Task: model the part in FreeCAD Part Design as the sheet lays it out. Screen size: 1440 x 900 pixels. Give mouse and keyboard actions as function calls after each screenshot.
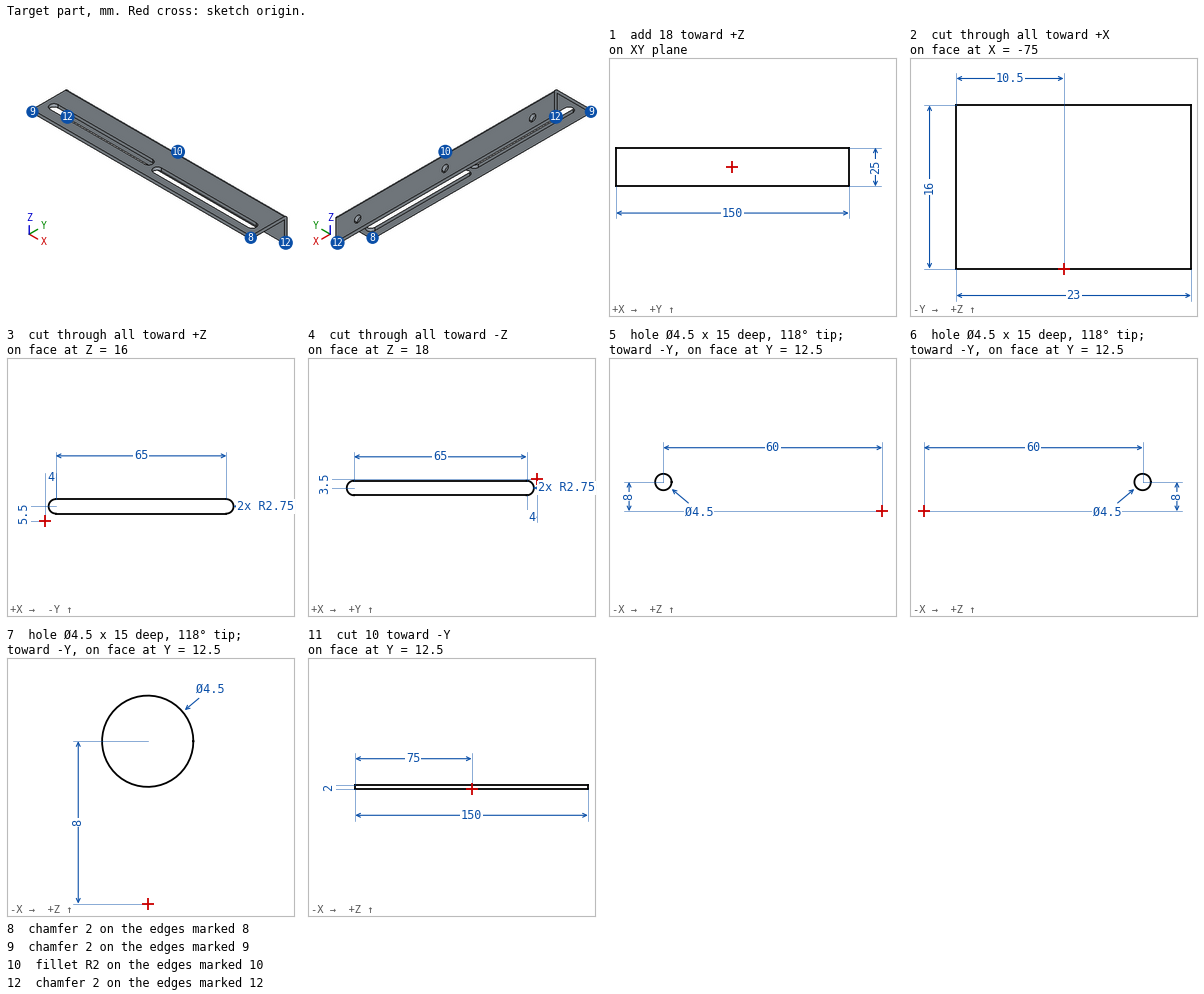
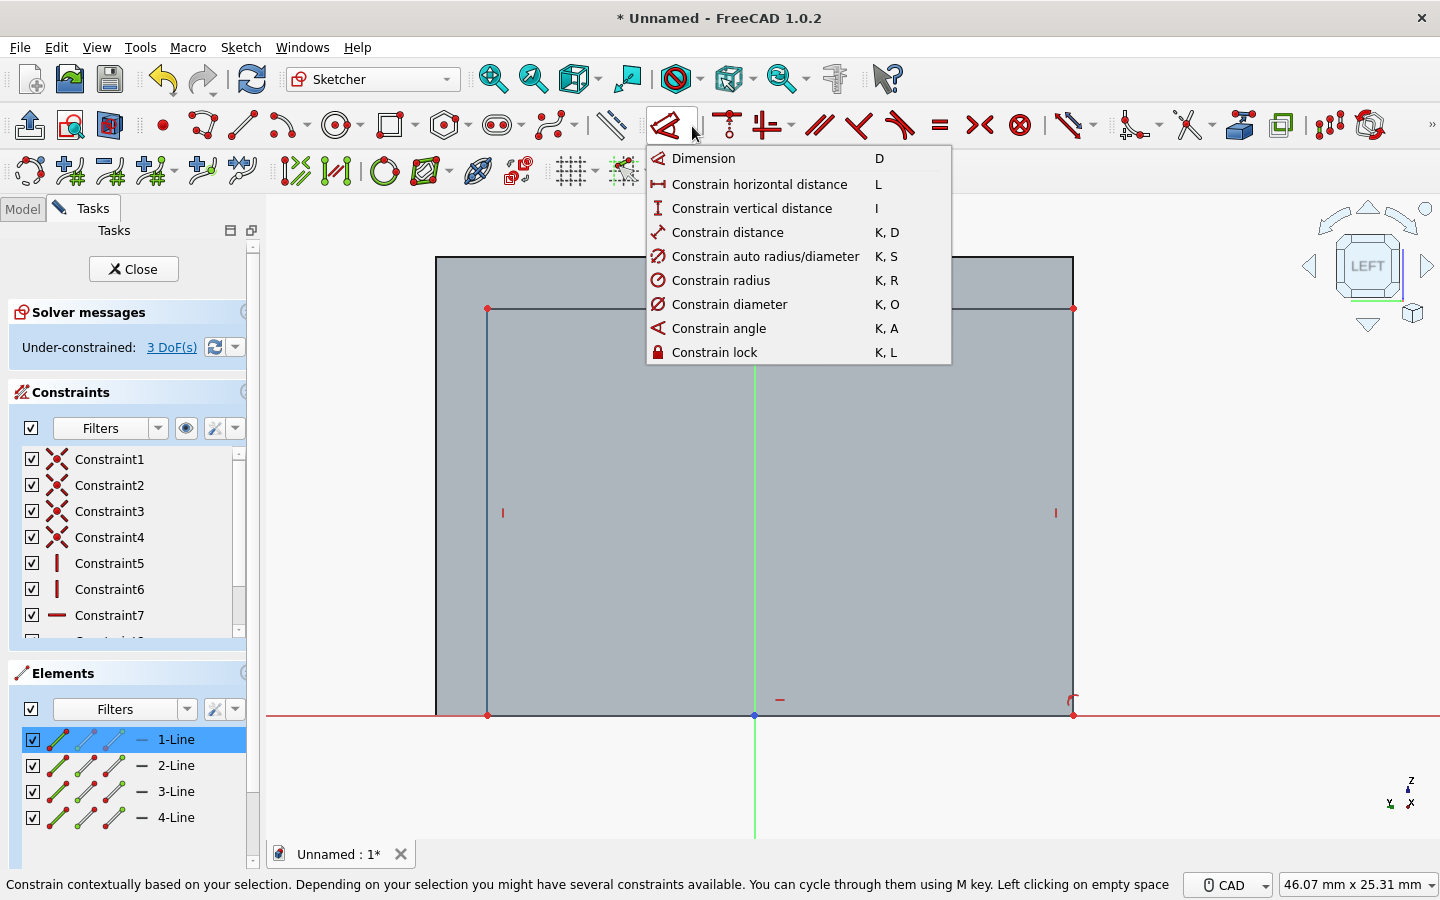
click(799, 208)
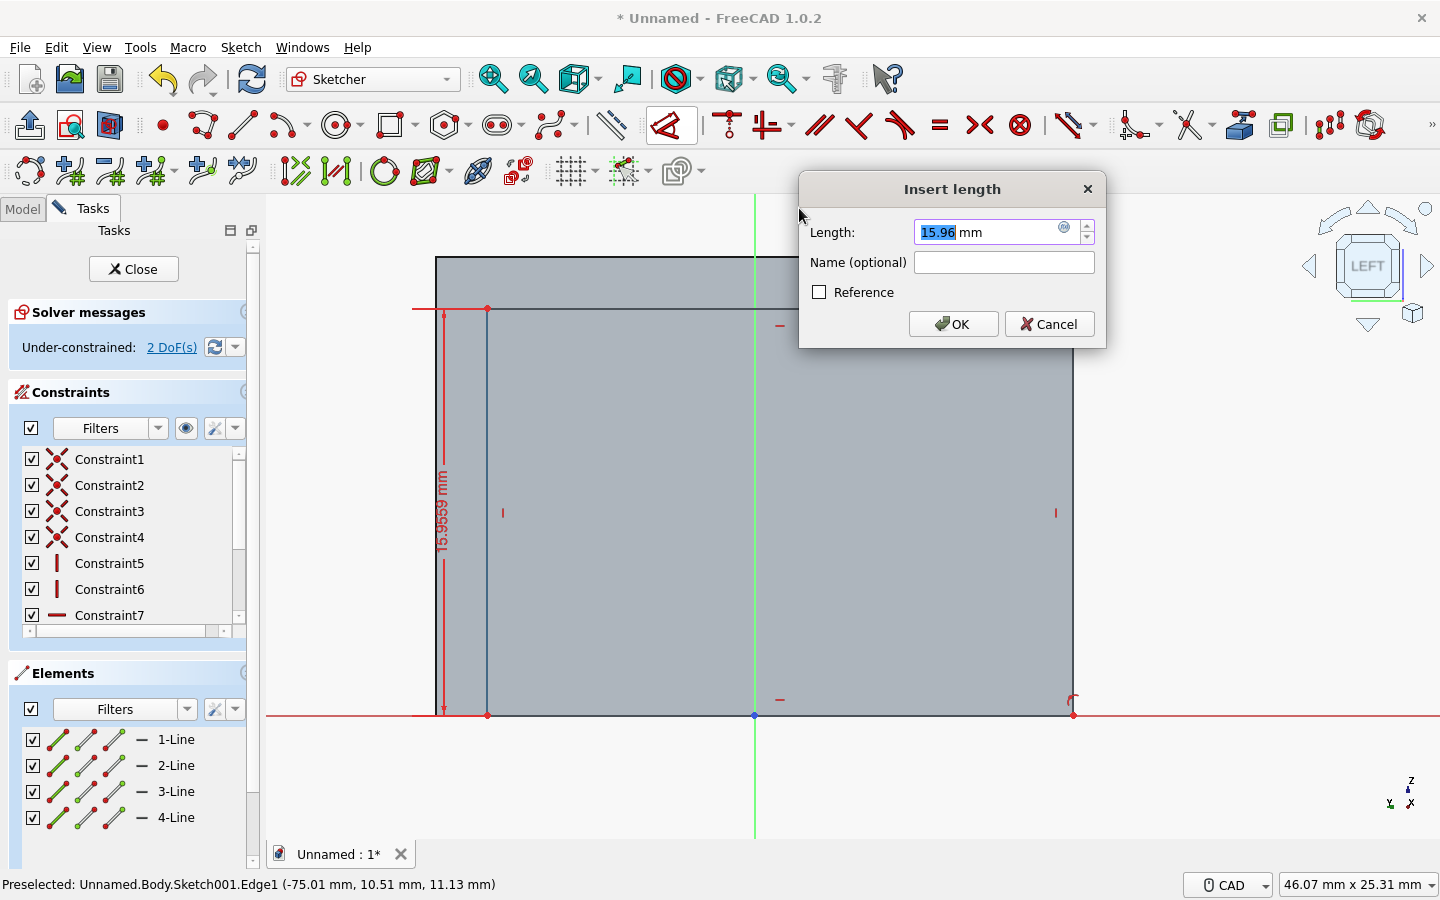
text(16)
key(Return)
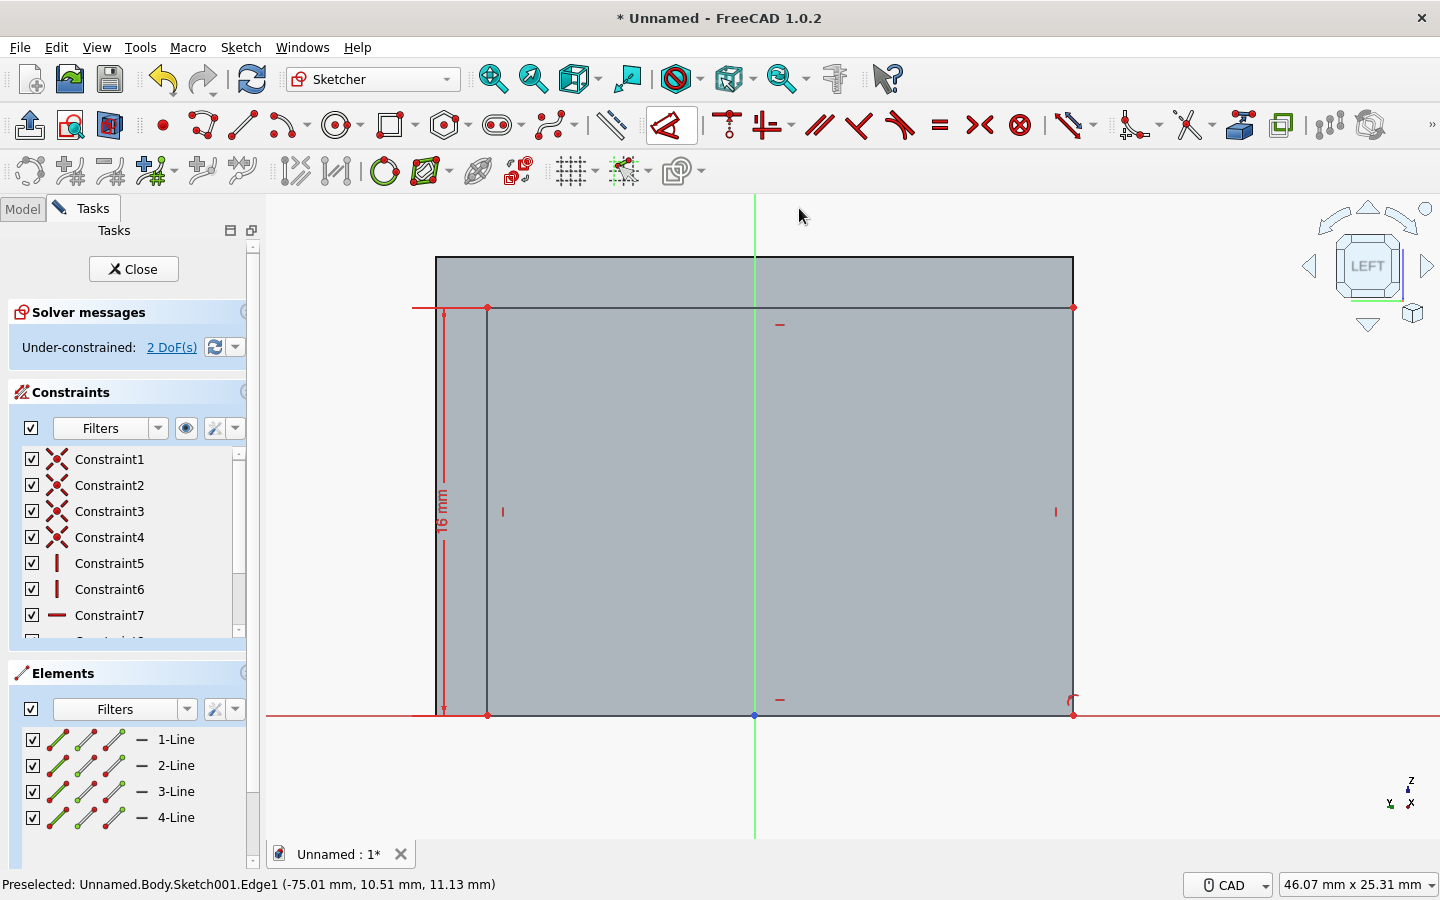
click(663, 716)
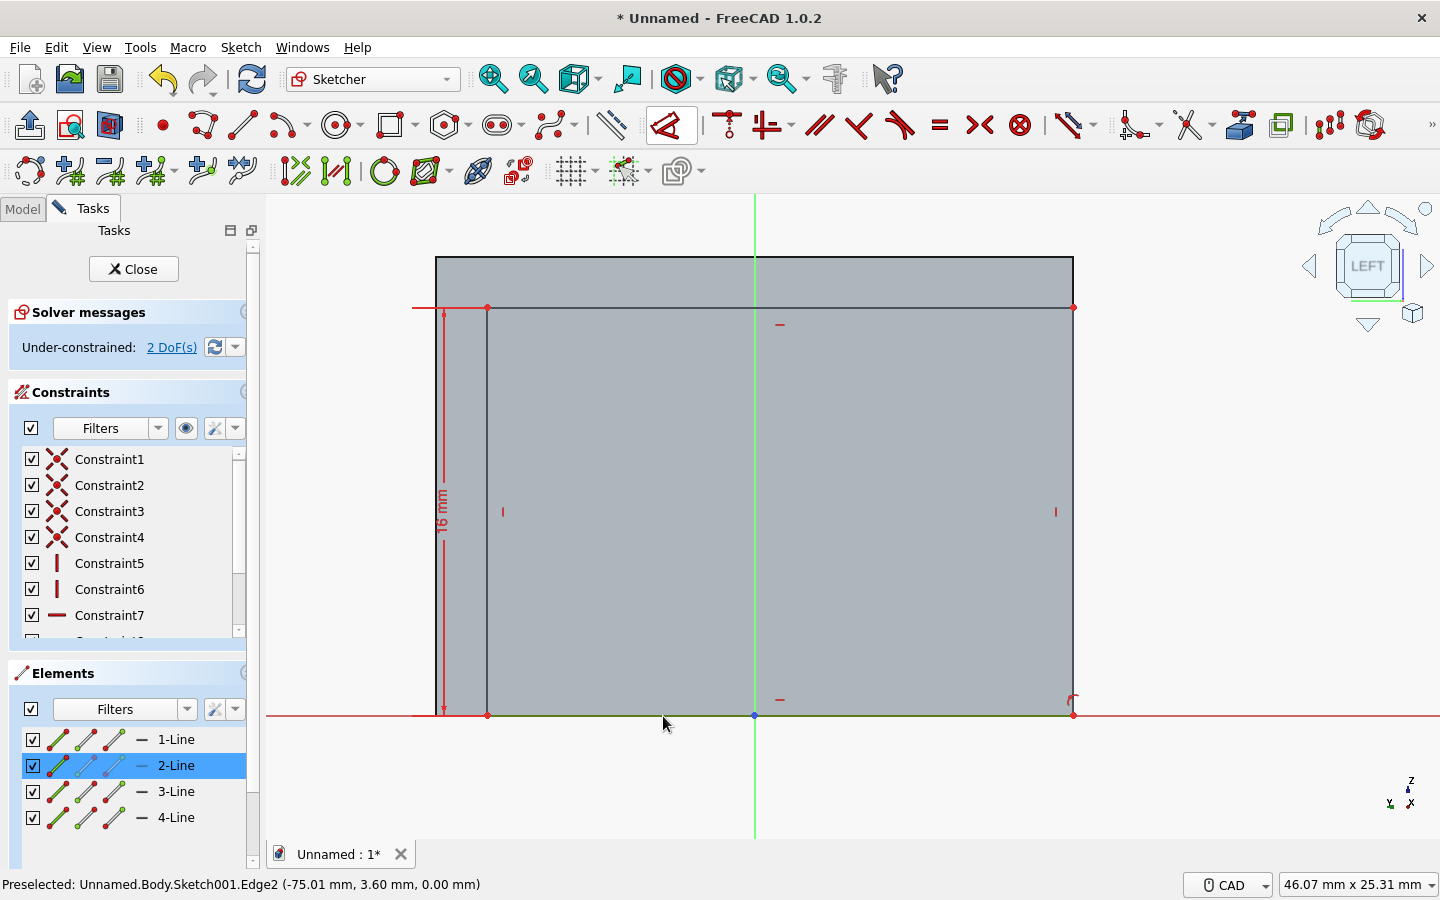
key(l)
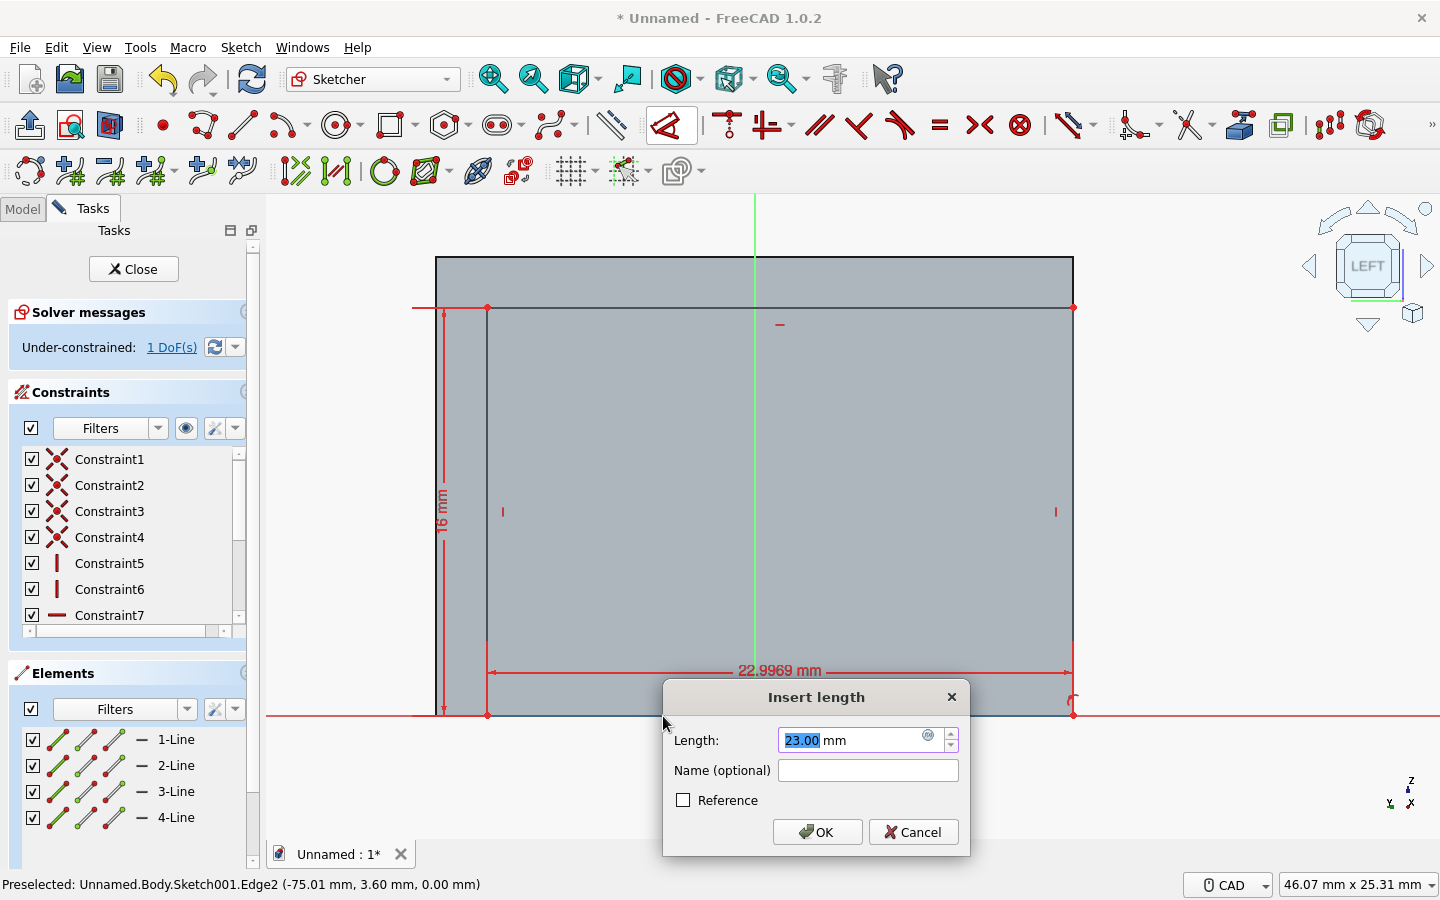
text(23)
key(Return)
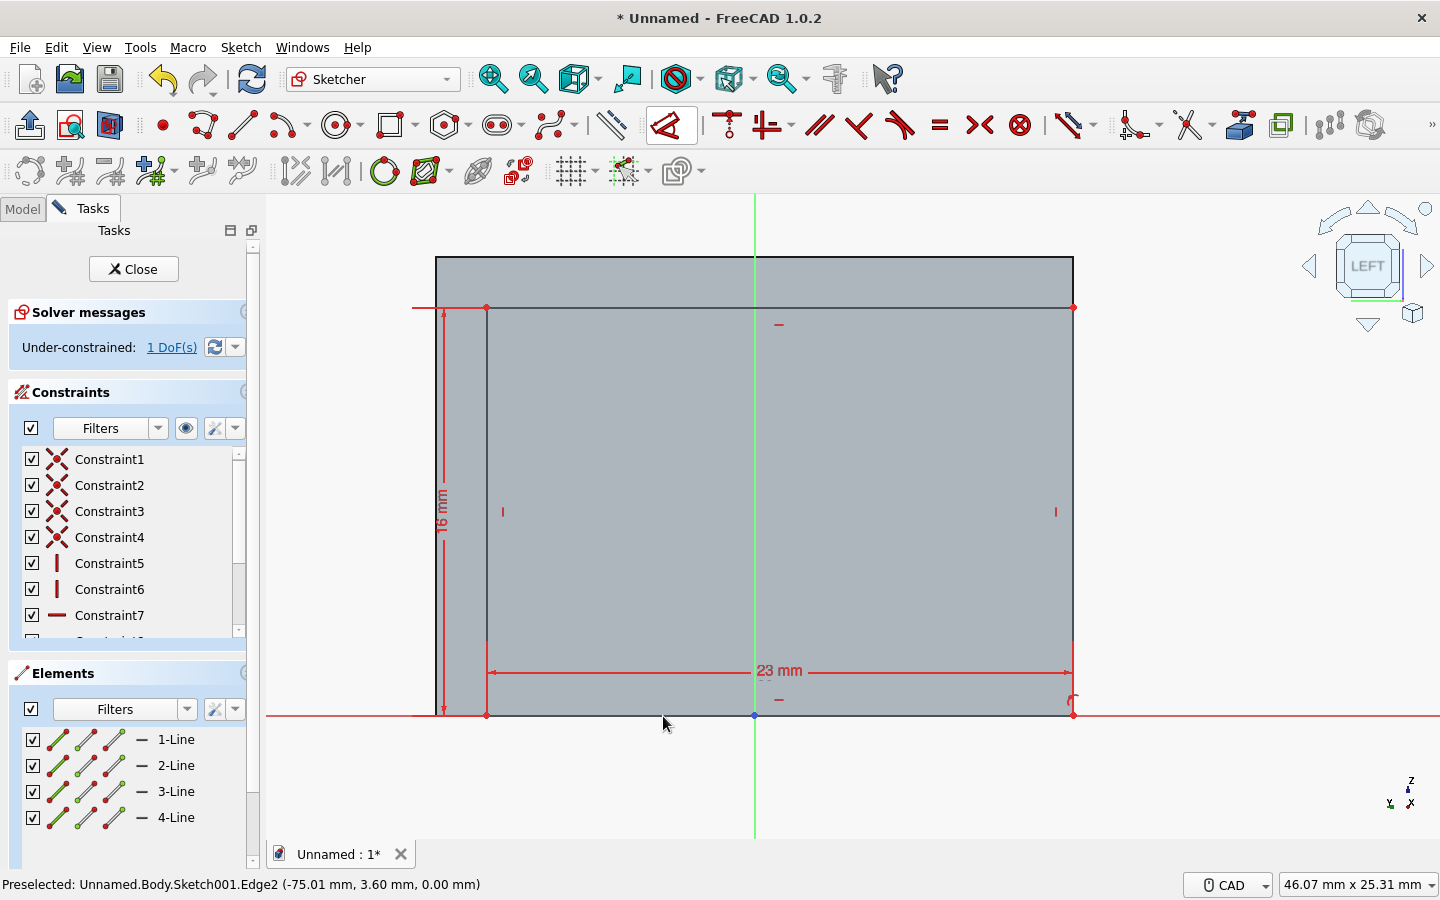
click(487, 308)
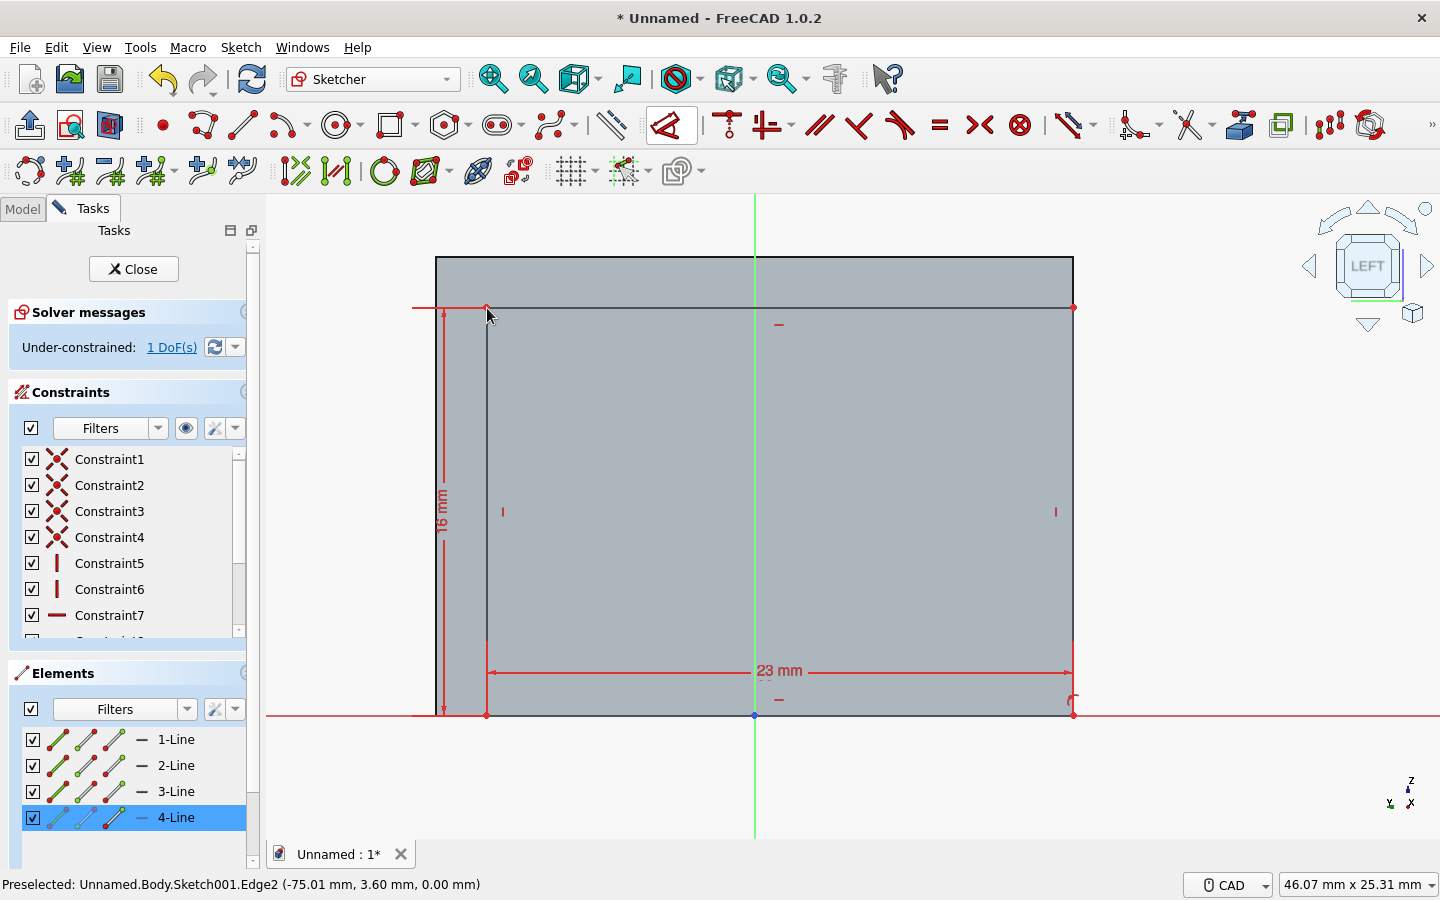
click(692, 126)